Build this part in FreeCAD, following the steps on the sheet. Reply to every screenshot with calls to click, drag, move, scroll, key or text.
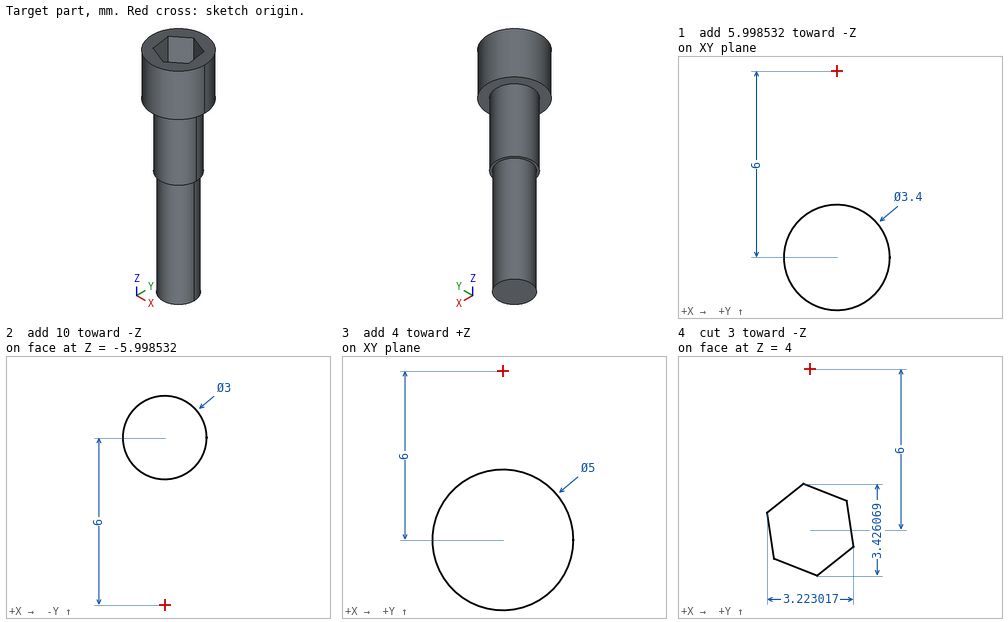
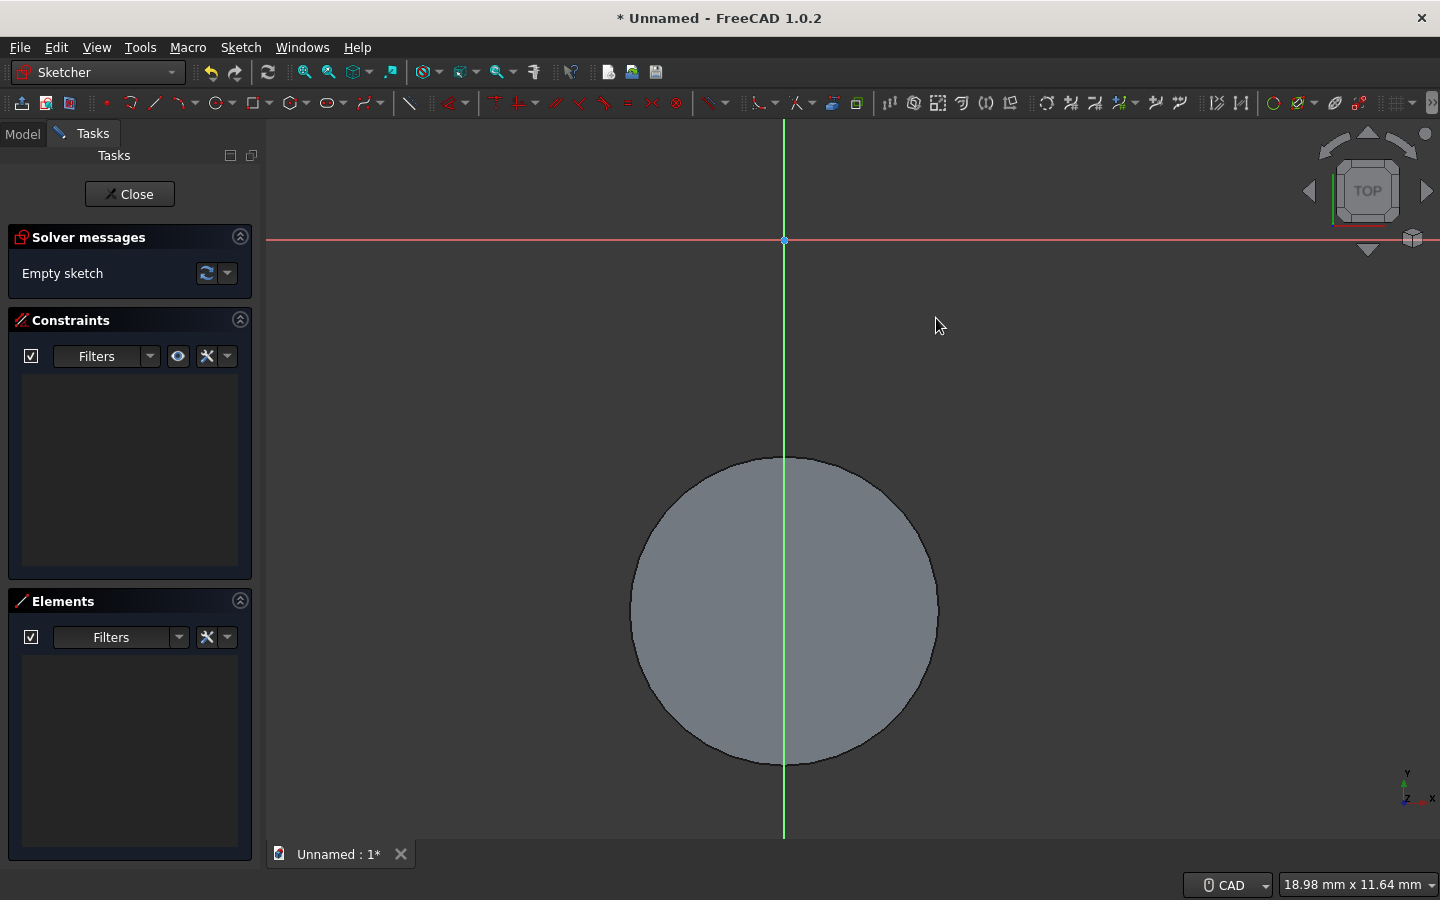
click(290, 104)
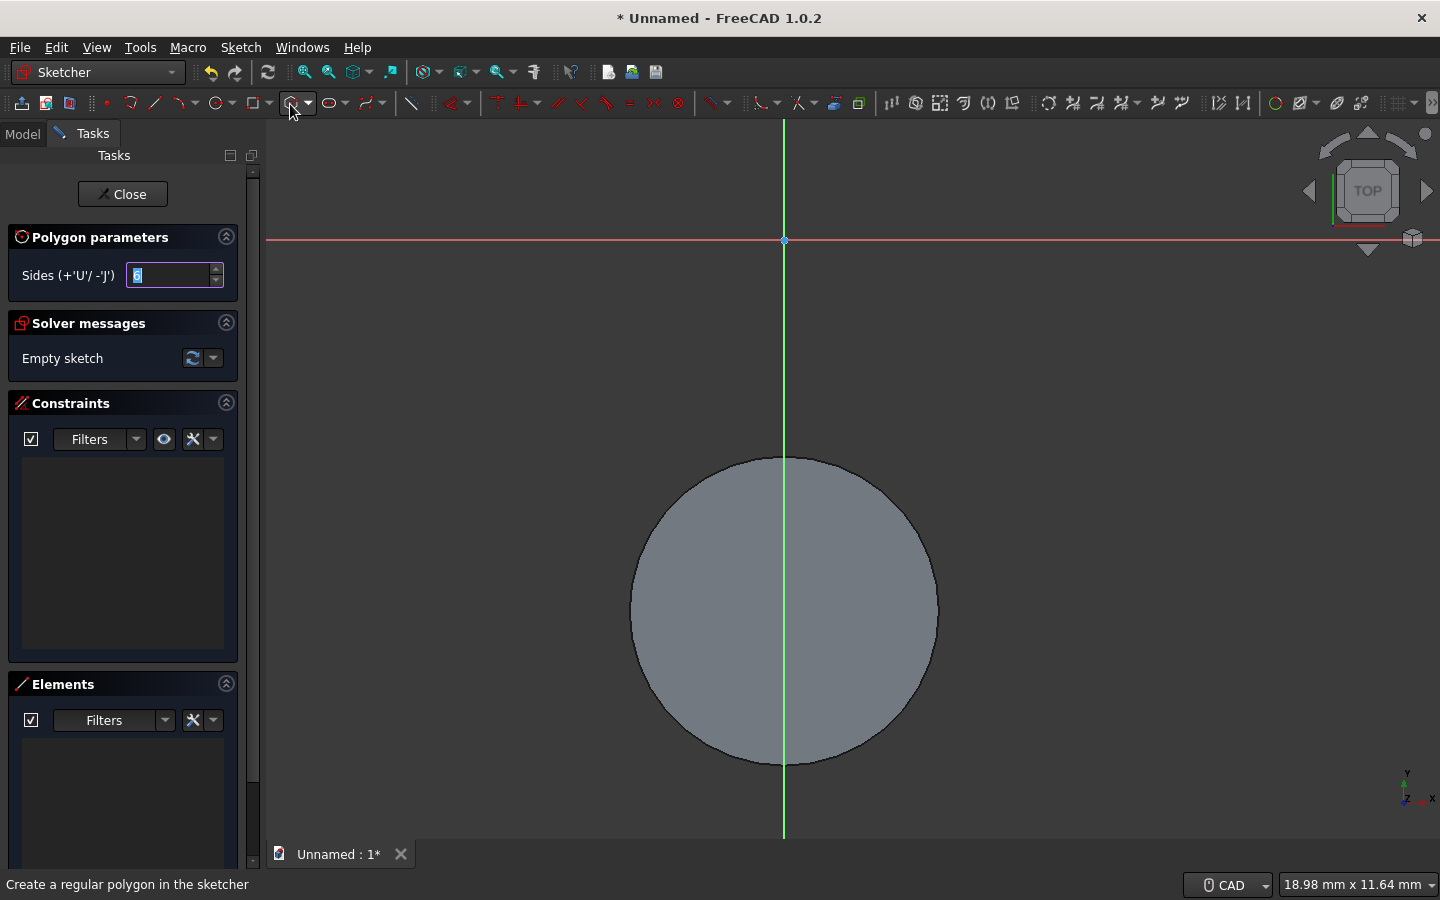
click(784, 611)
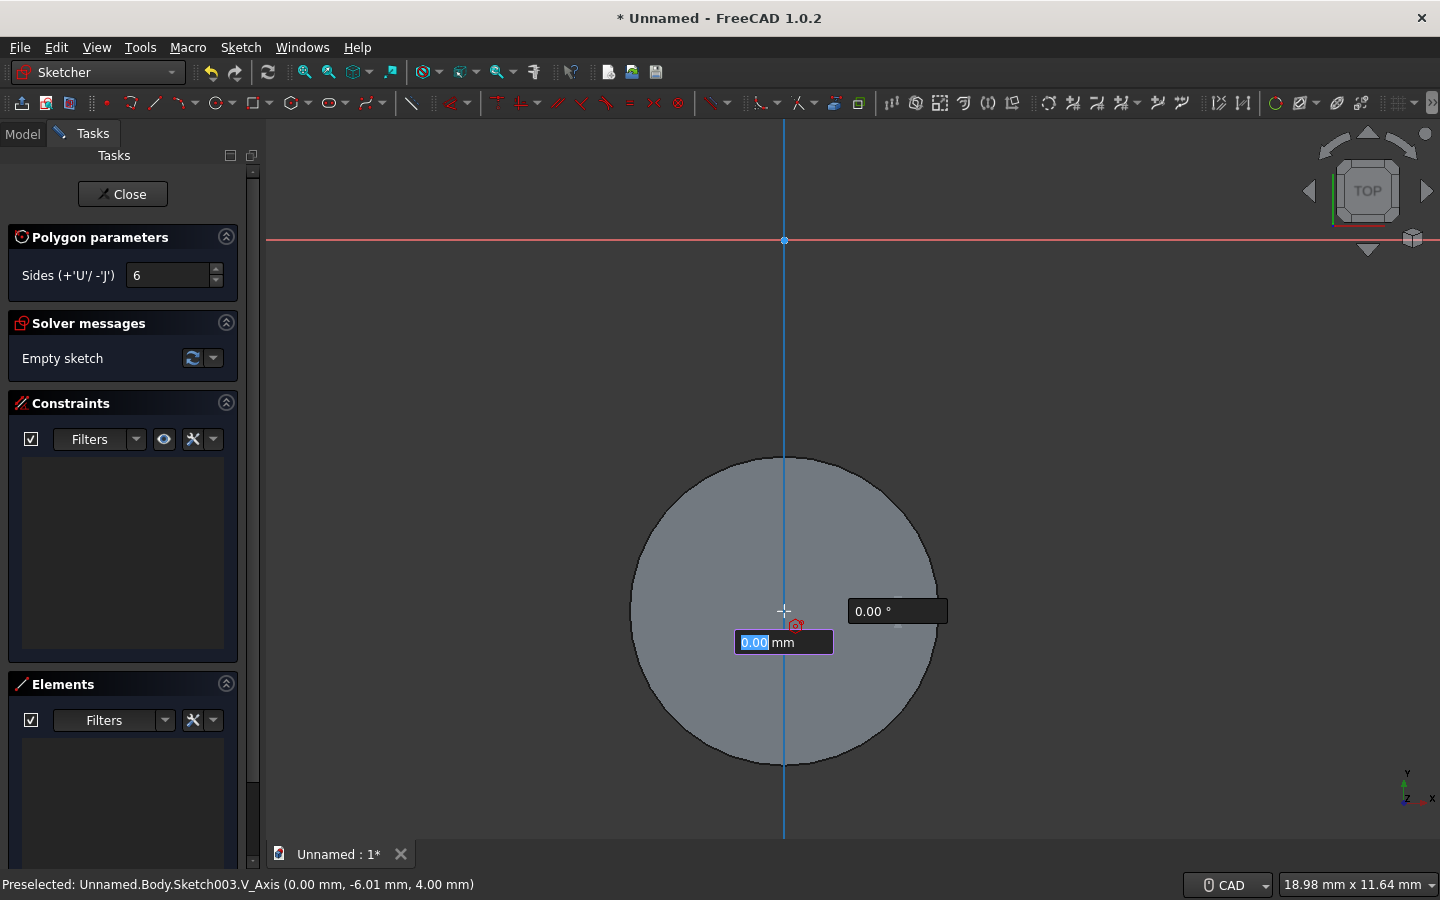
click(685, 572)
right_click(685, 572)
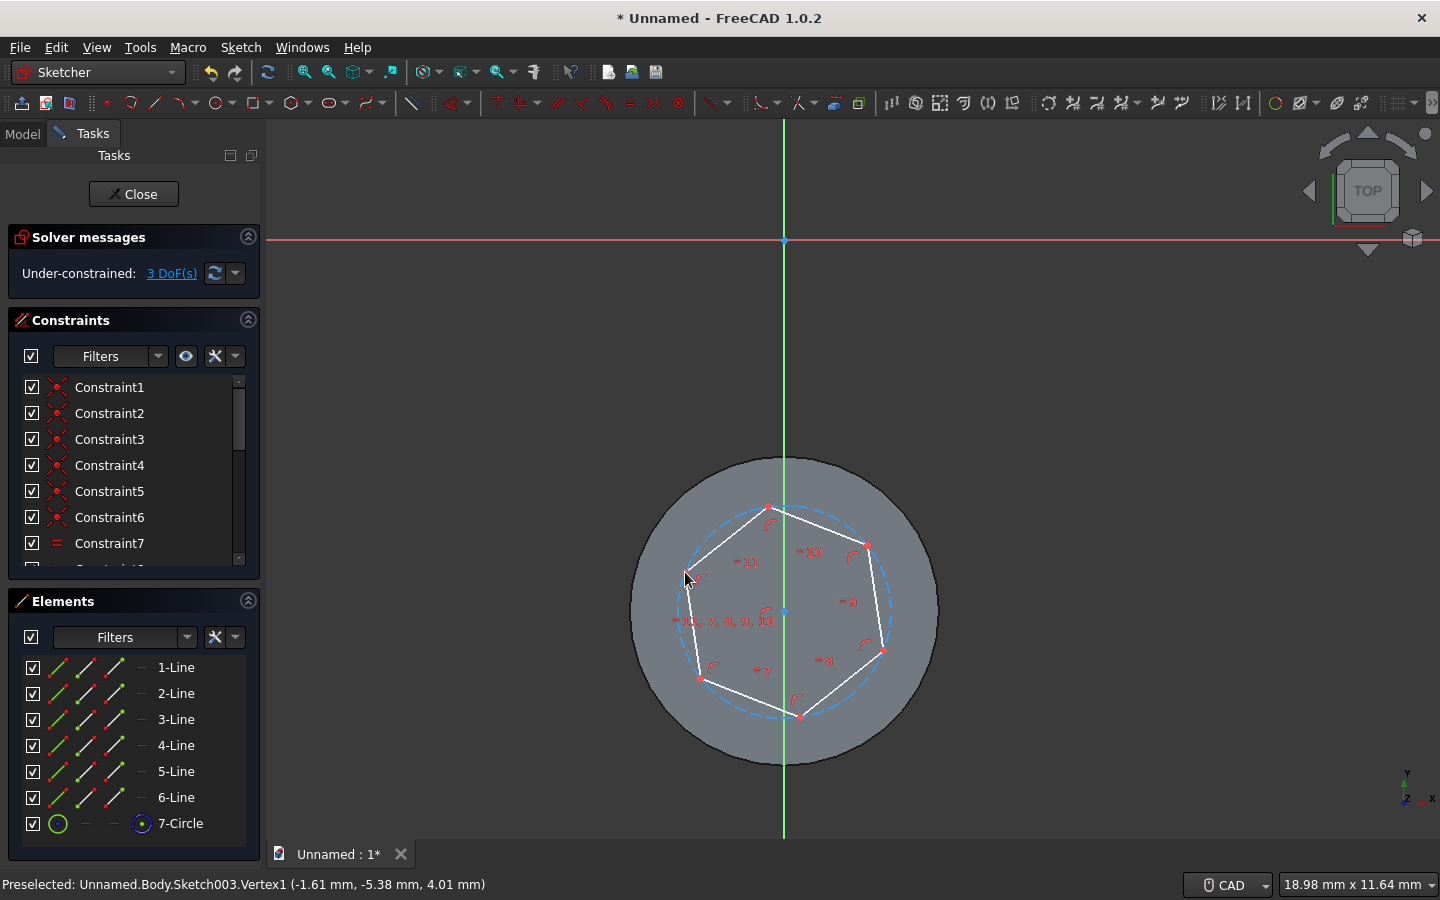
key(d)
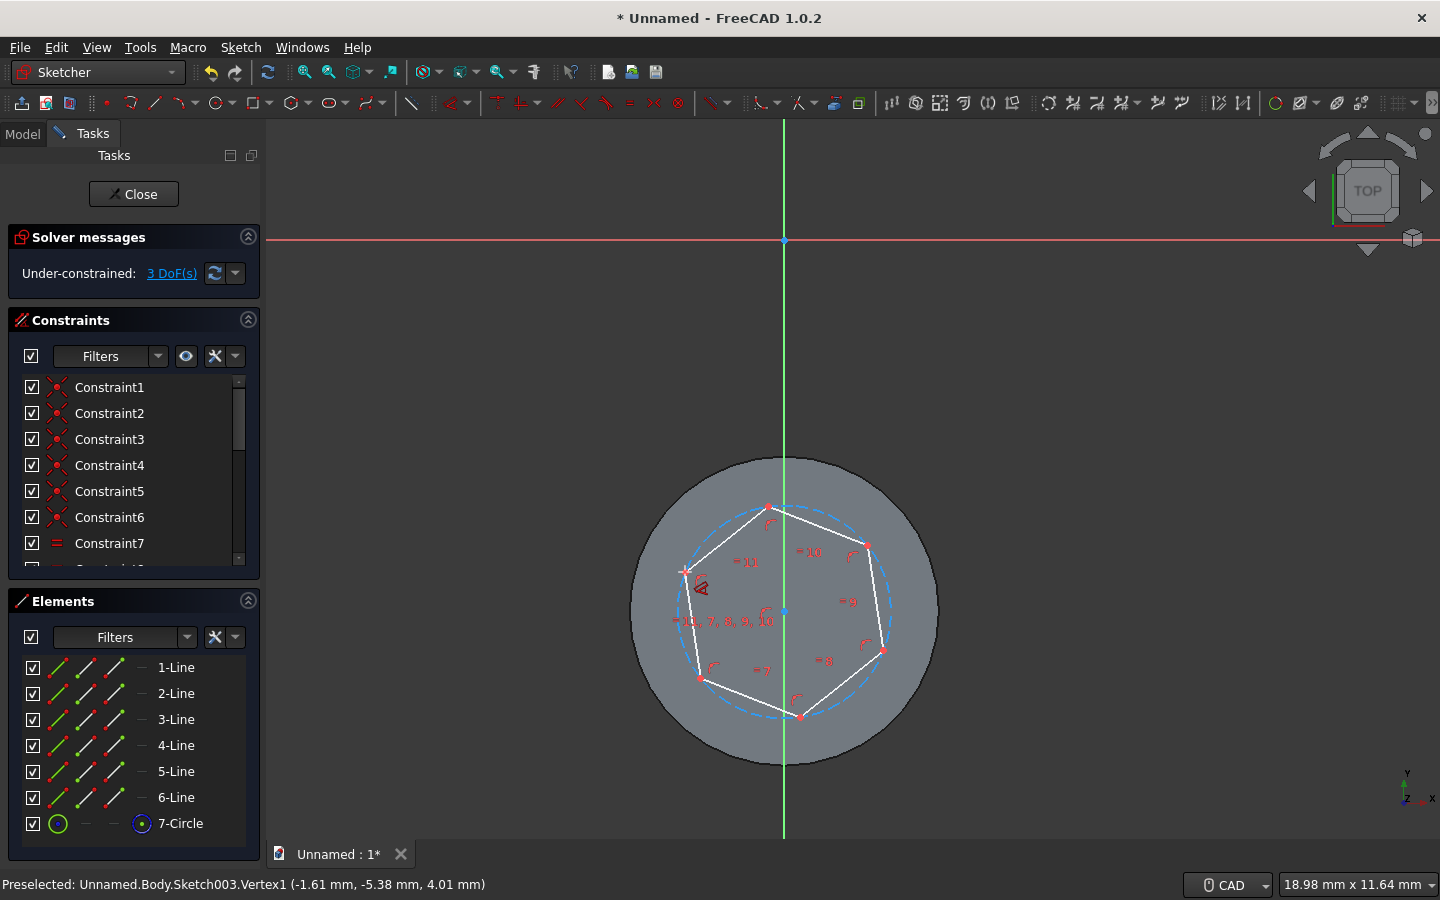
click(784, 612)
click(818, 426)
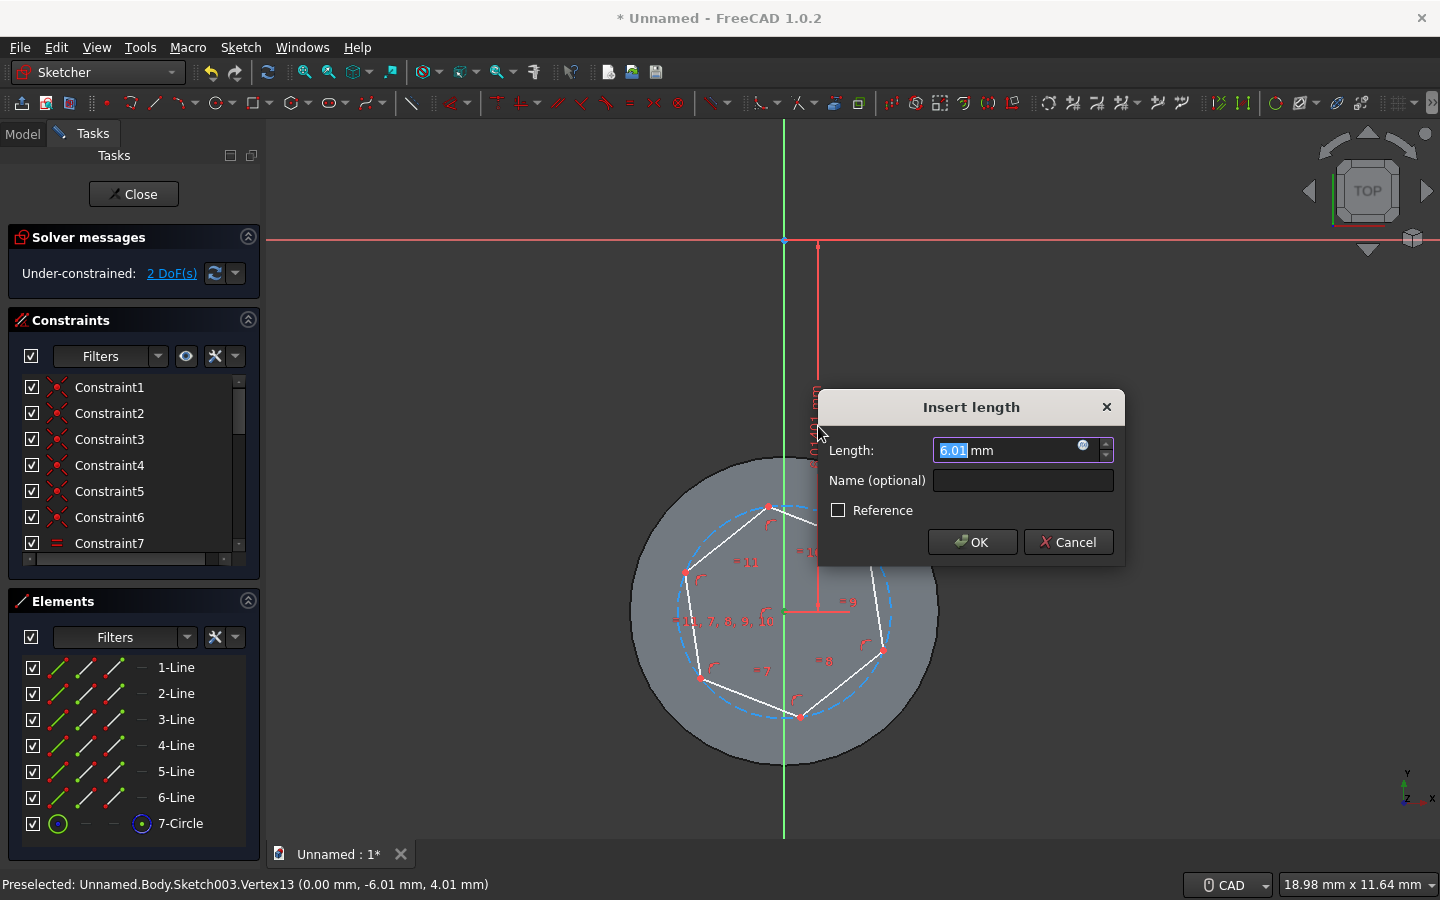
text(6)
key(Return)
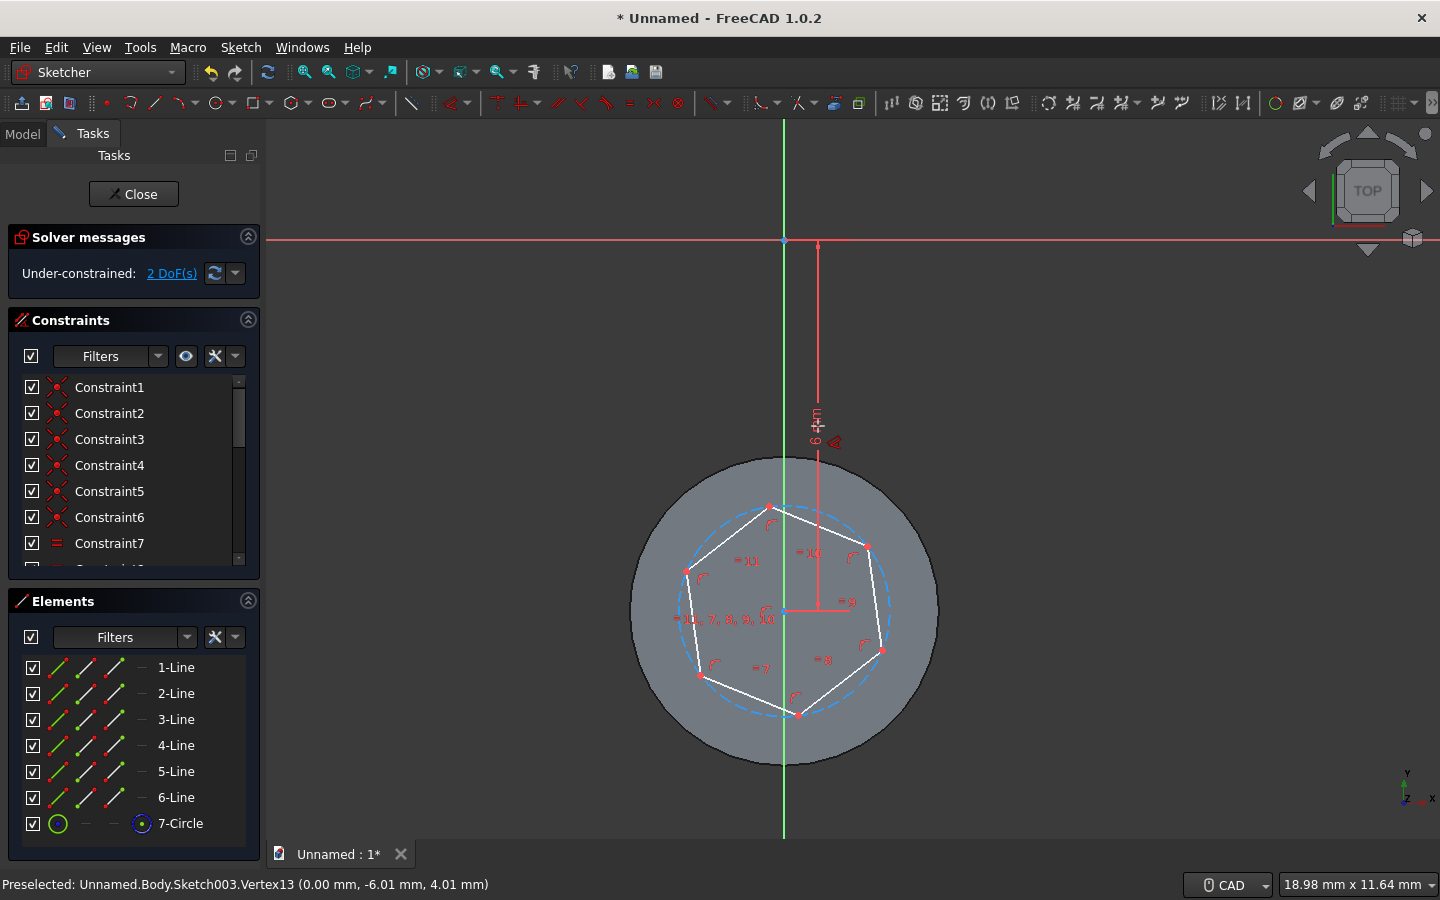
click(687, 571)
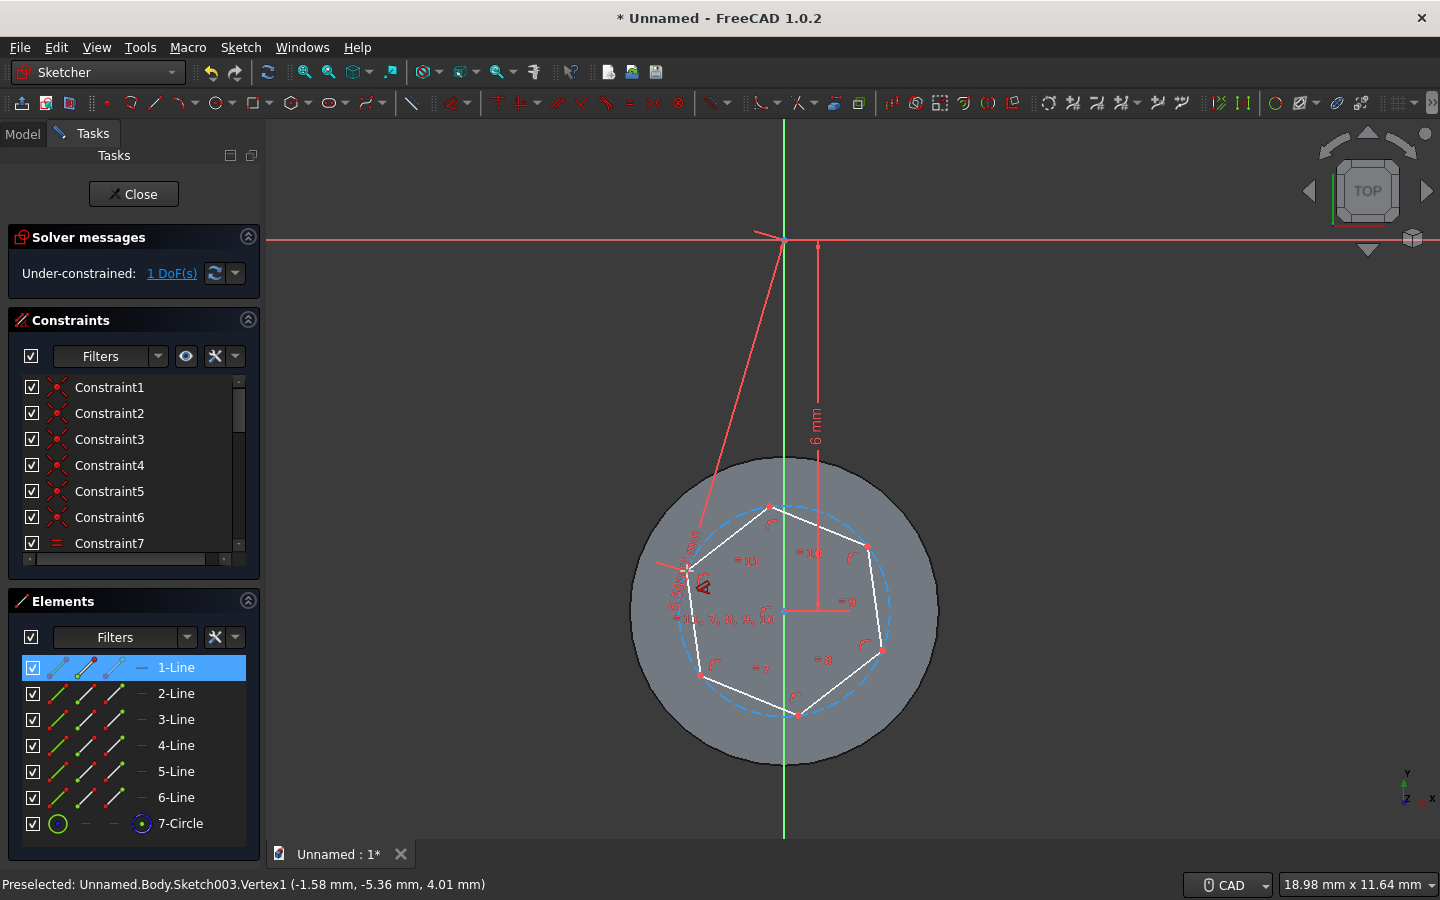
click(882, 651)
click(716, 709)